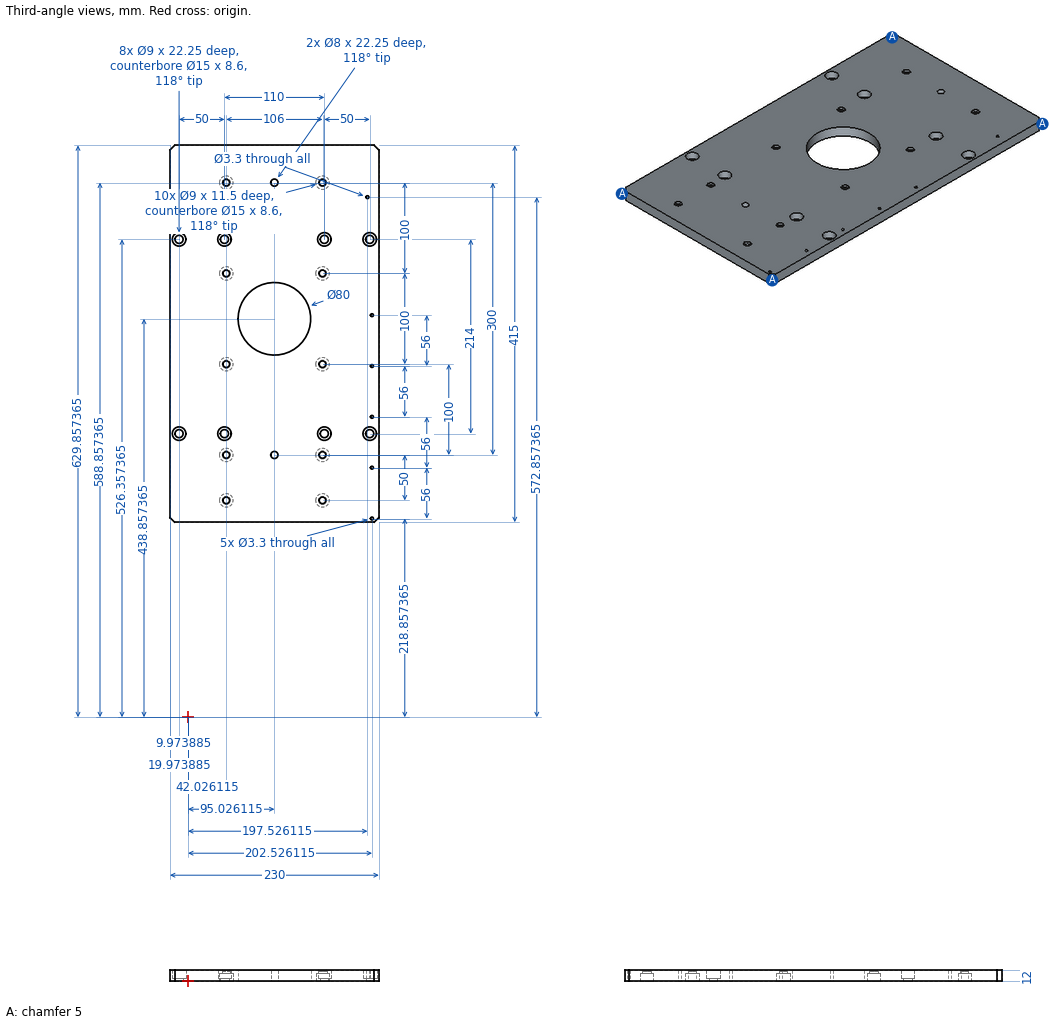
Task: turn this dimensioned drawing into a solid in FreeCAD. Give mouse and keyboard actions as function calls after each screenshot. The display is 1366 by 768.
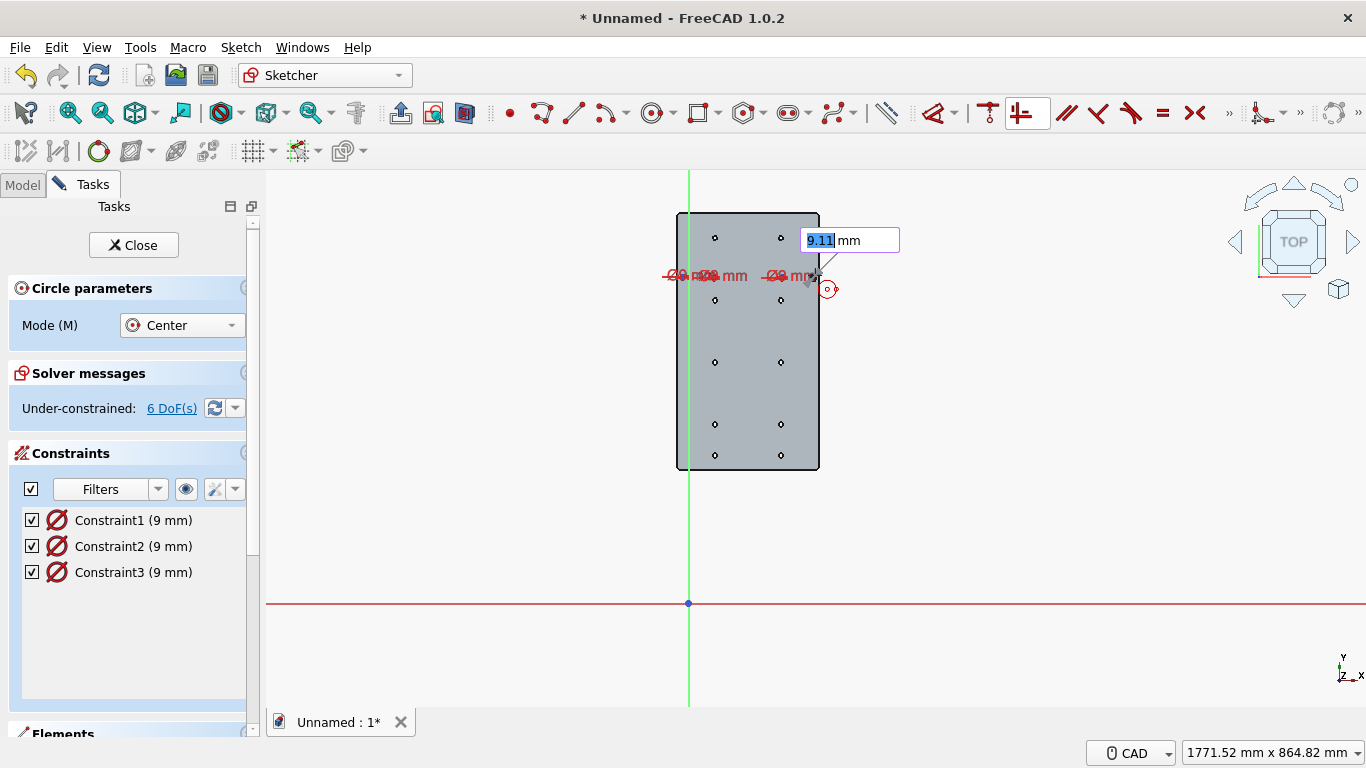
text(9)
key(Return)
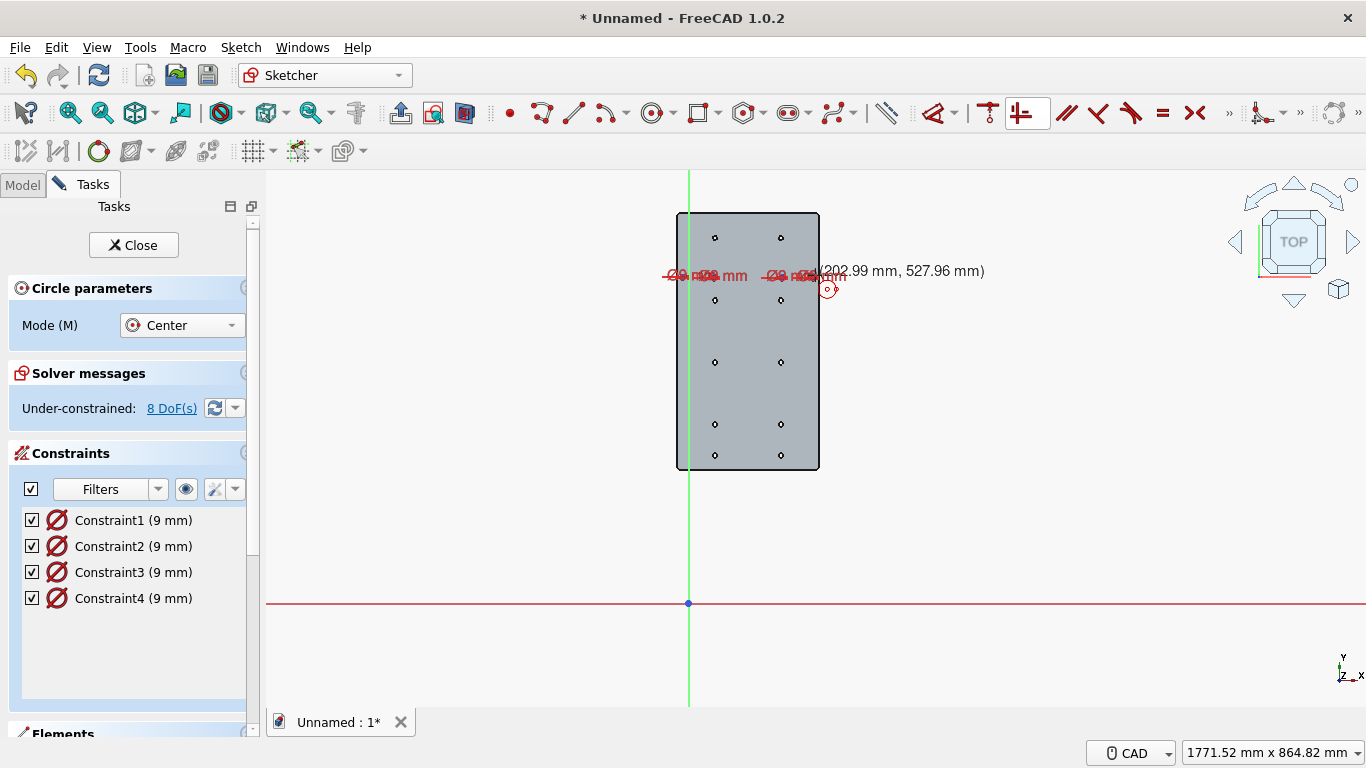
scroll(813, 410, up, 11)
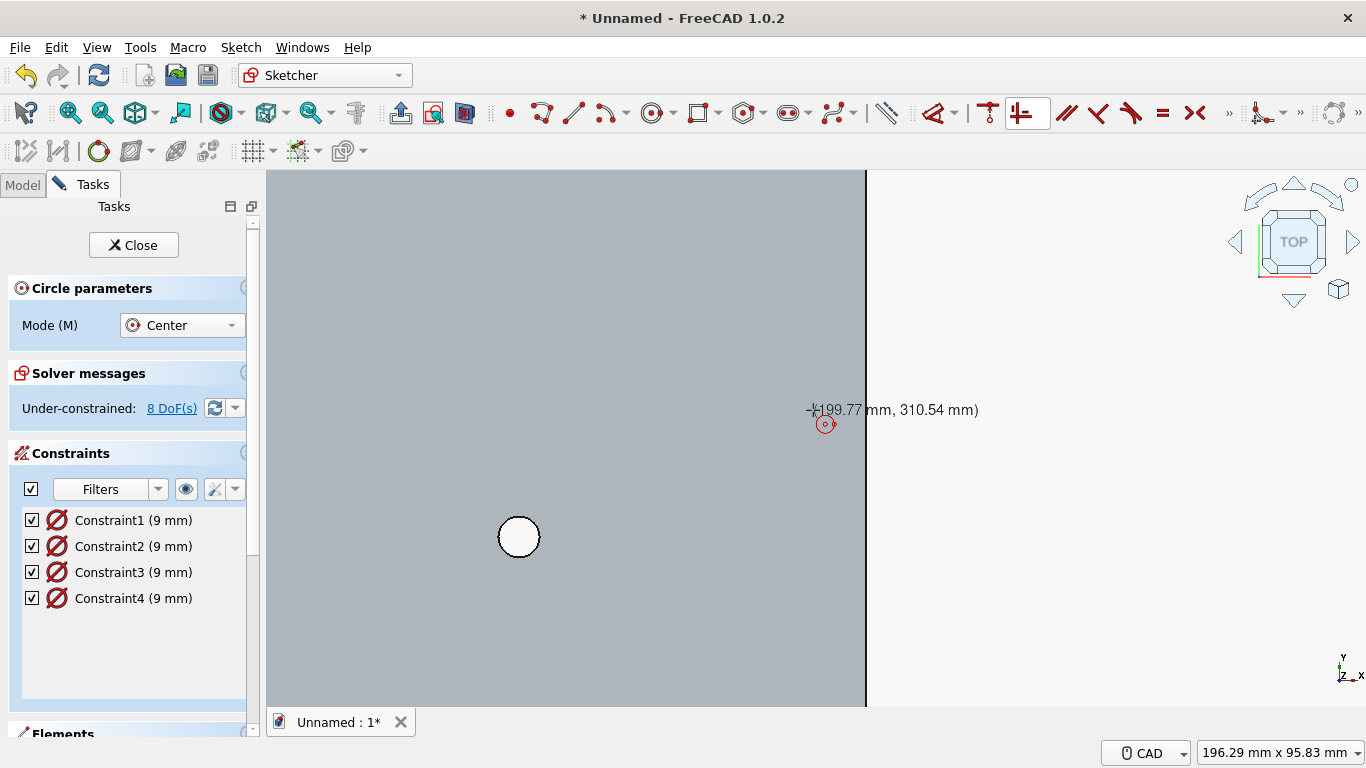
scroll(813, 410, down, 11)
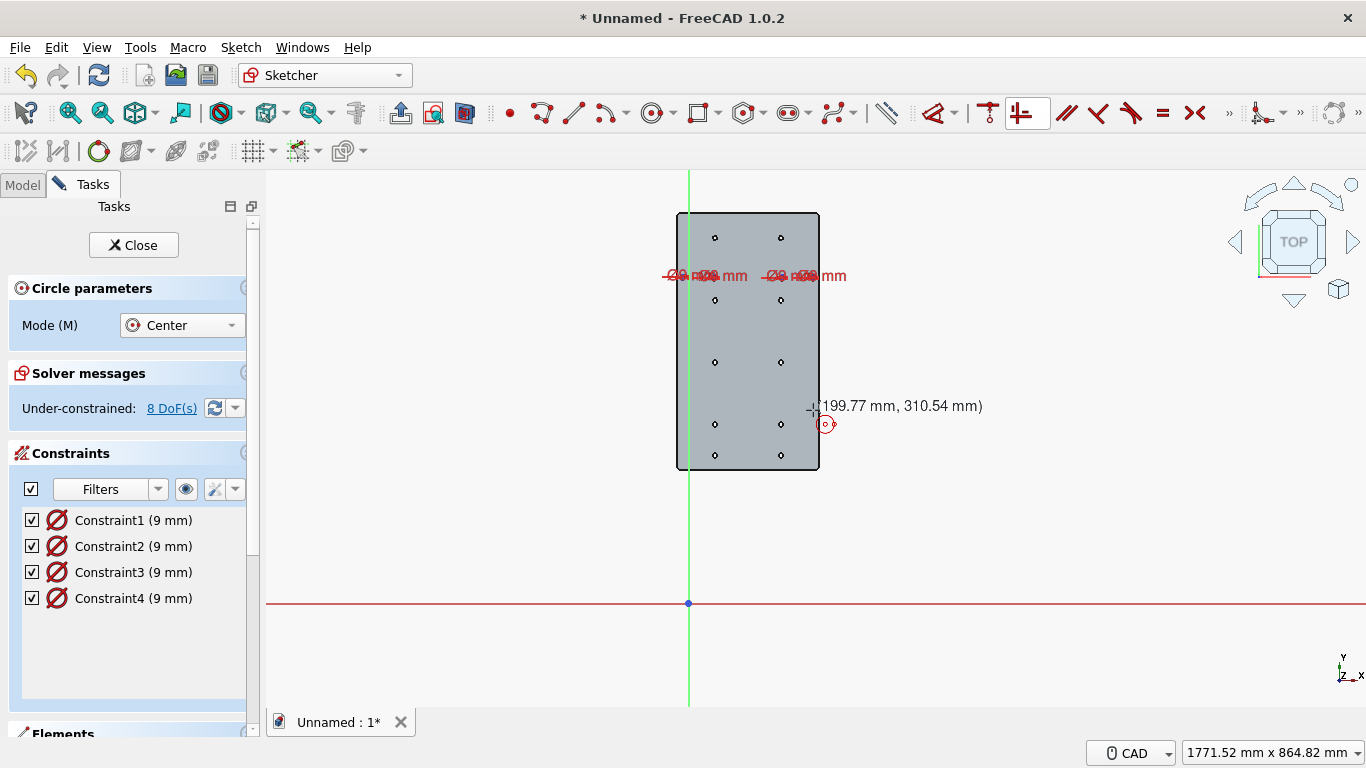
click(813, 410)
move(815, 408)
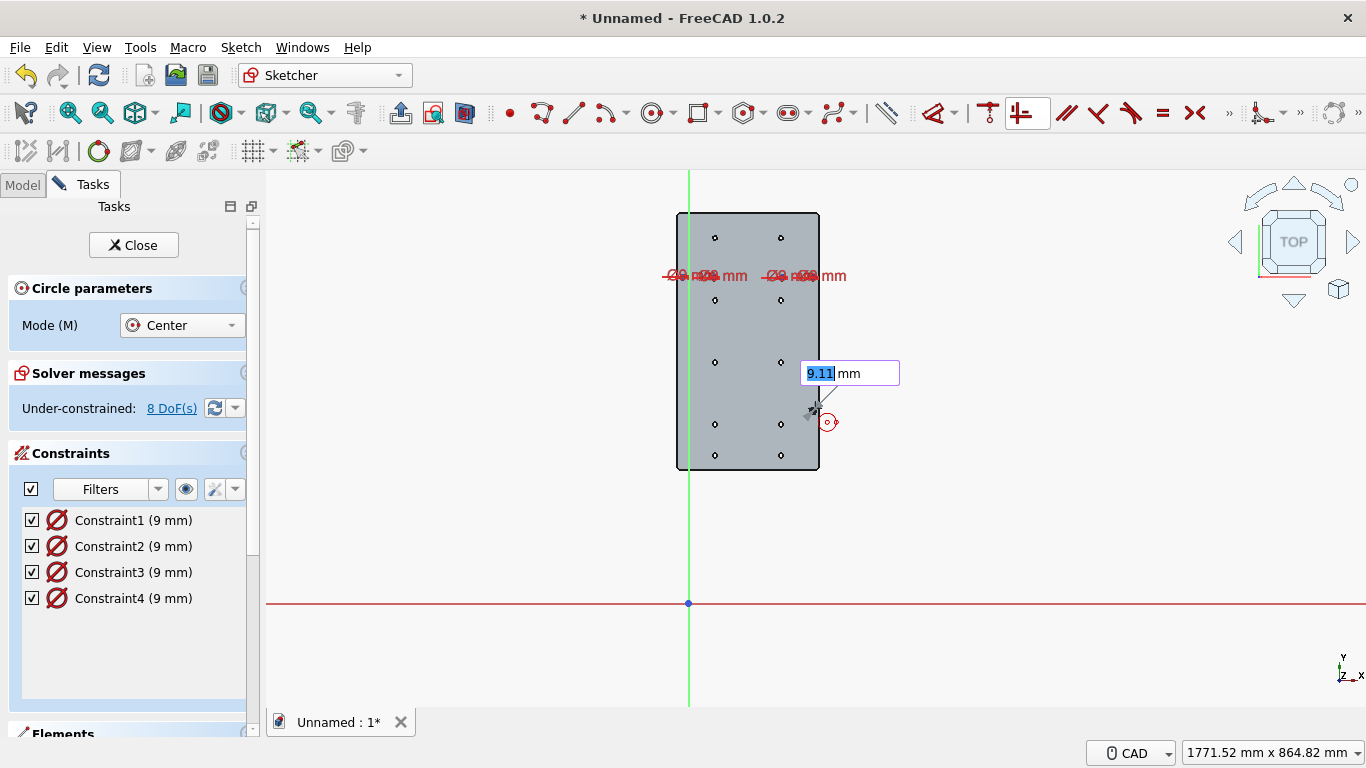
text(9)
key(Return)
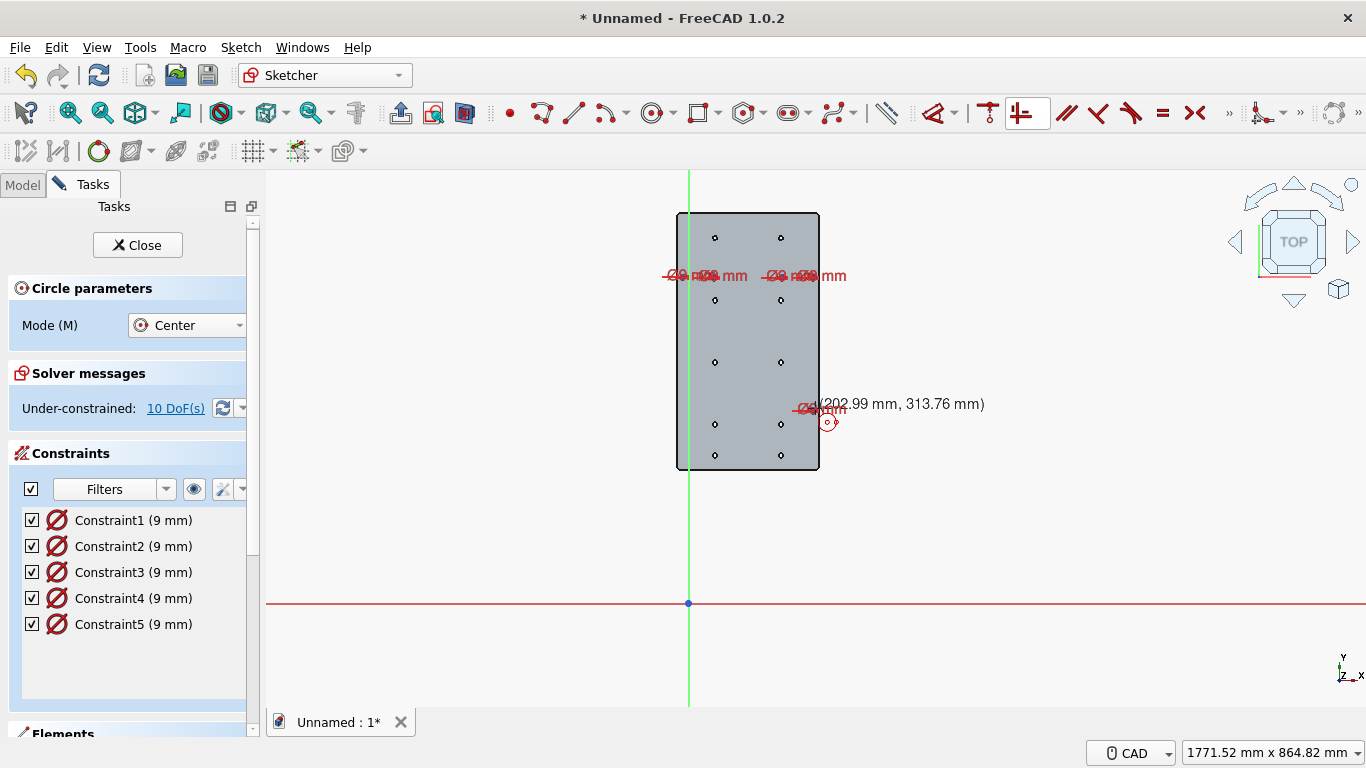
scroll(782, 410, up, 11)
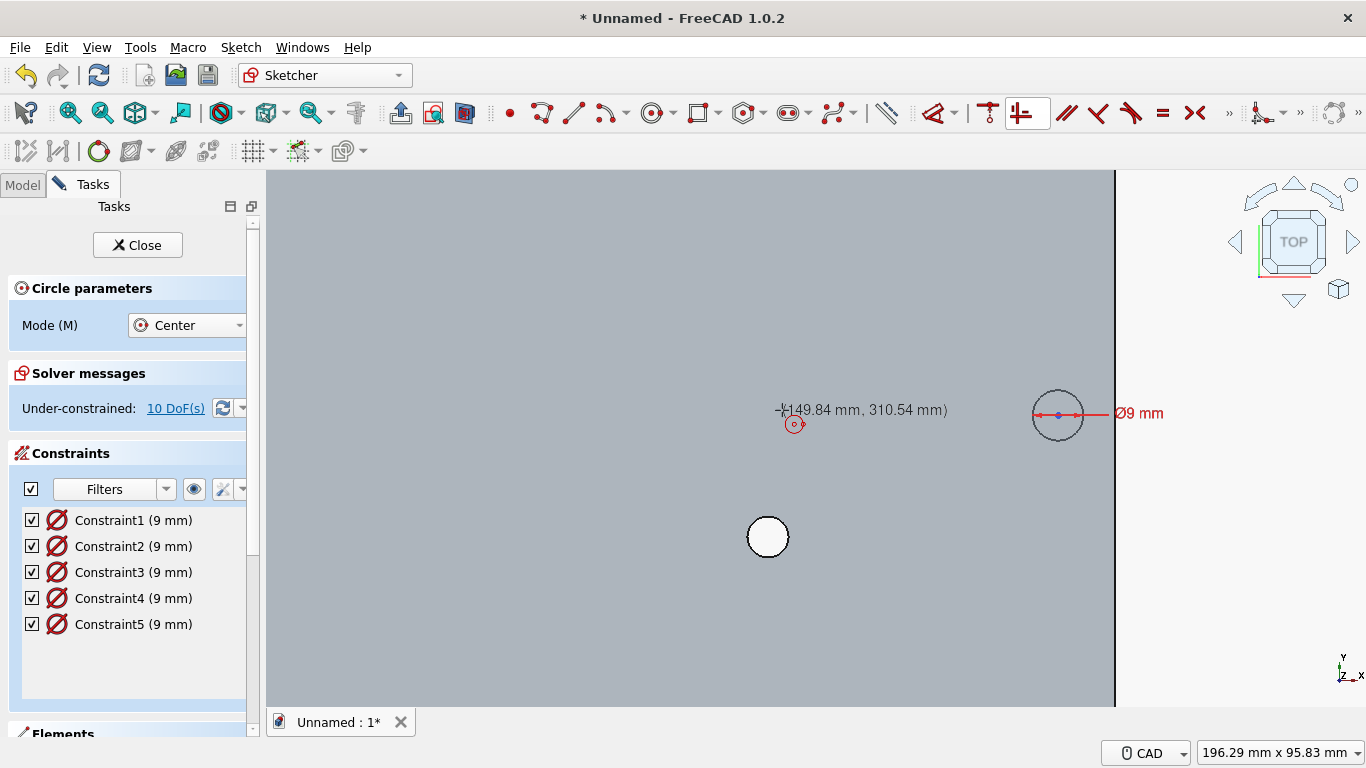
scroll(782, 410, down, 11)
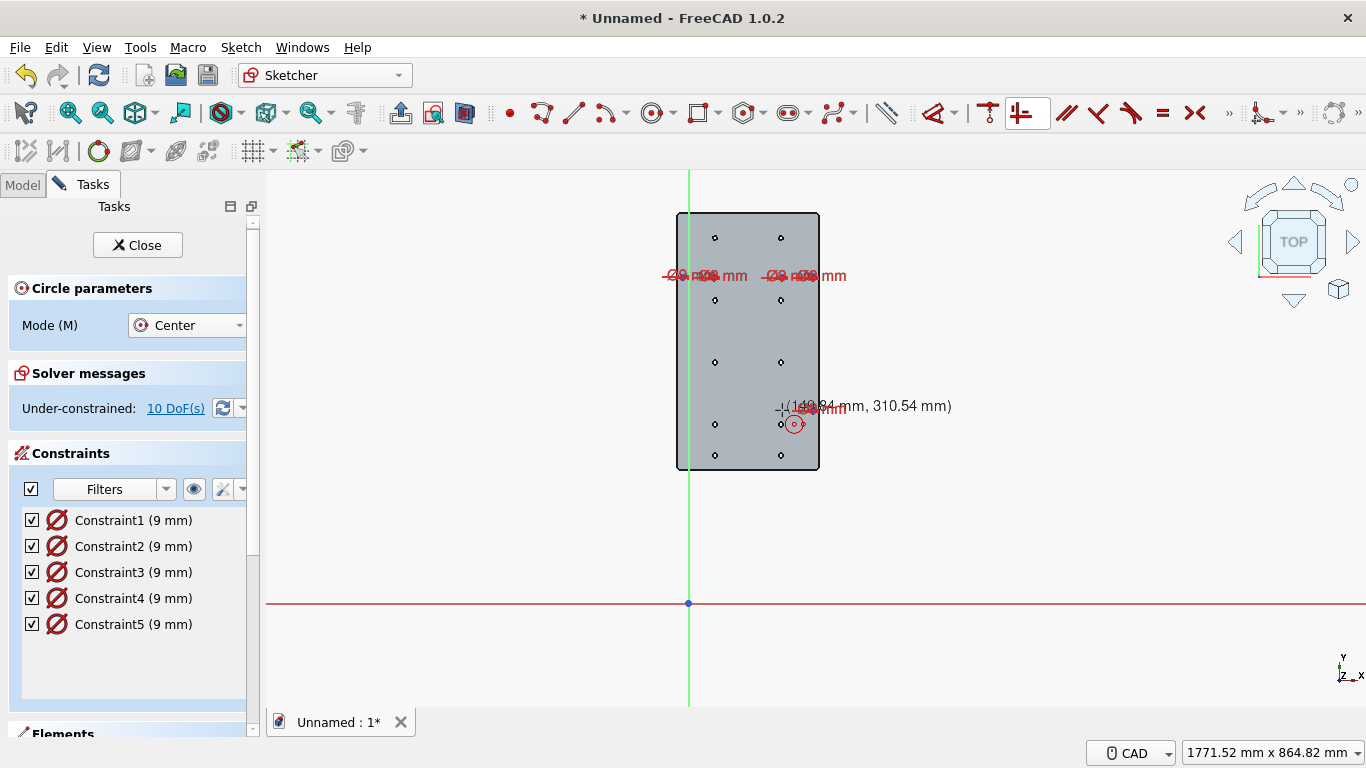
click(782, 410)
move(784, 408)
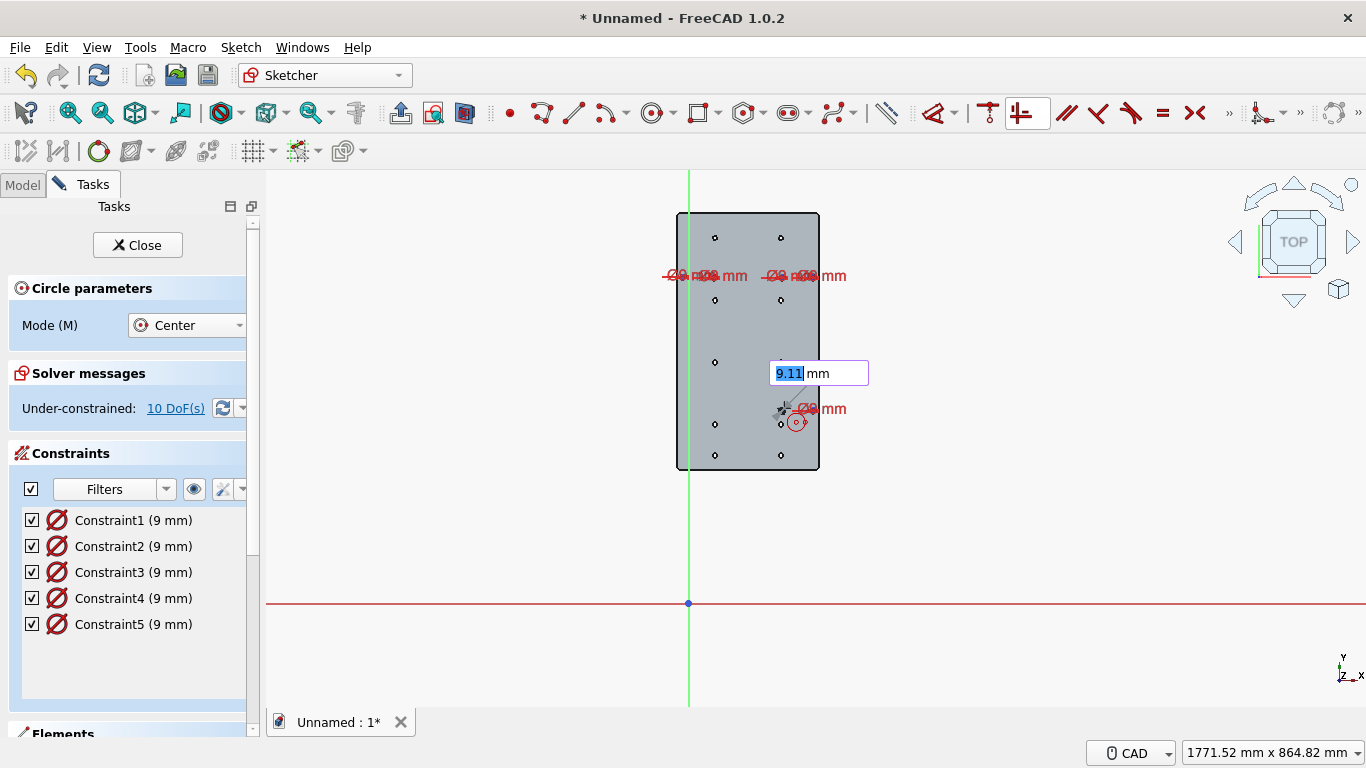
text(9)
key(Return)